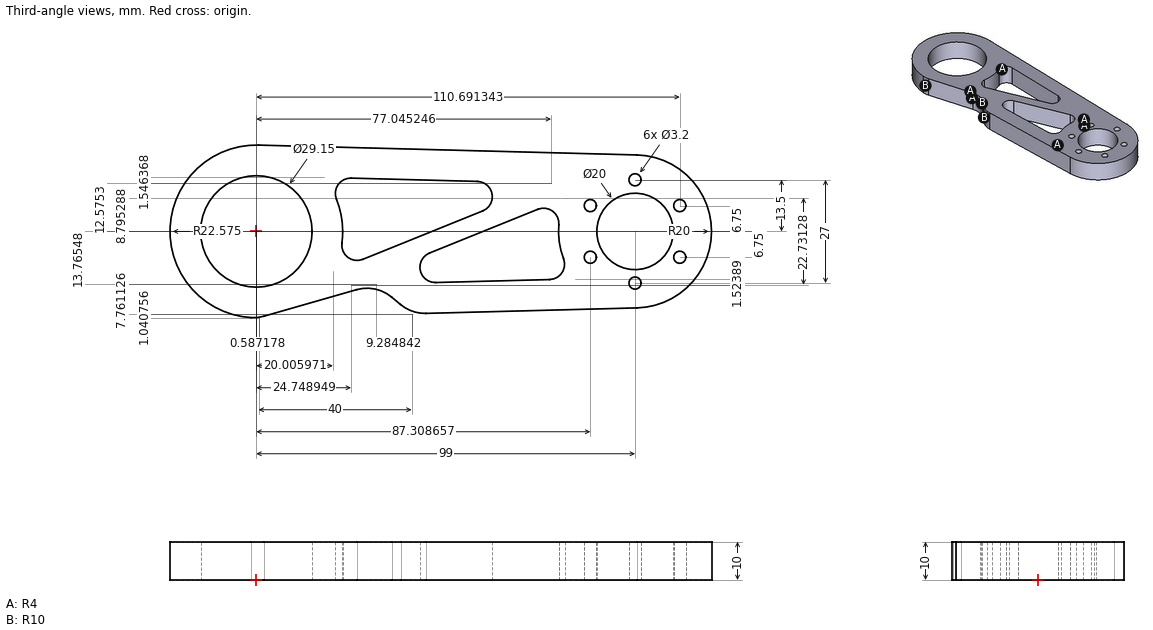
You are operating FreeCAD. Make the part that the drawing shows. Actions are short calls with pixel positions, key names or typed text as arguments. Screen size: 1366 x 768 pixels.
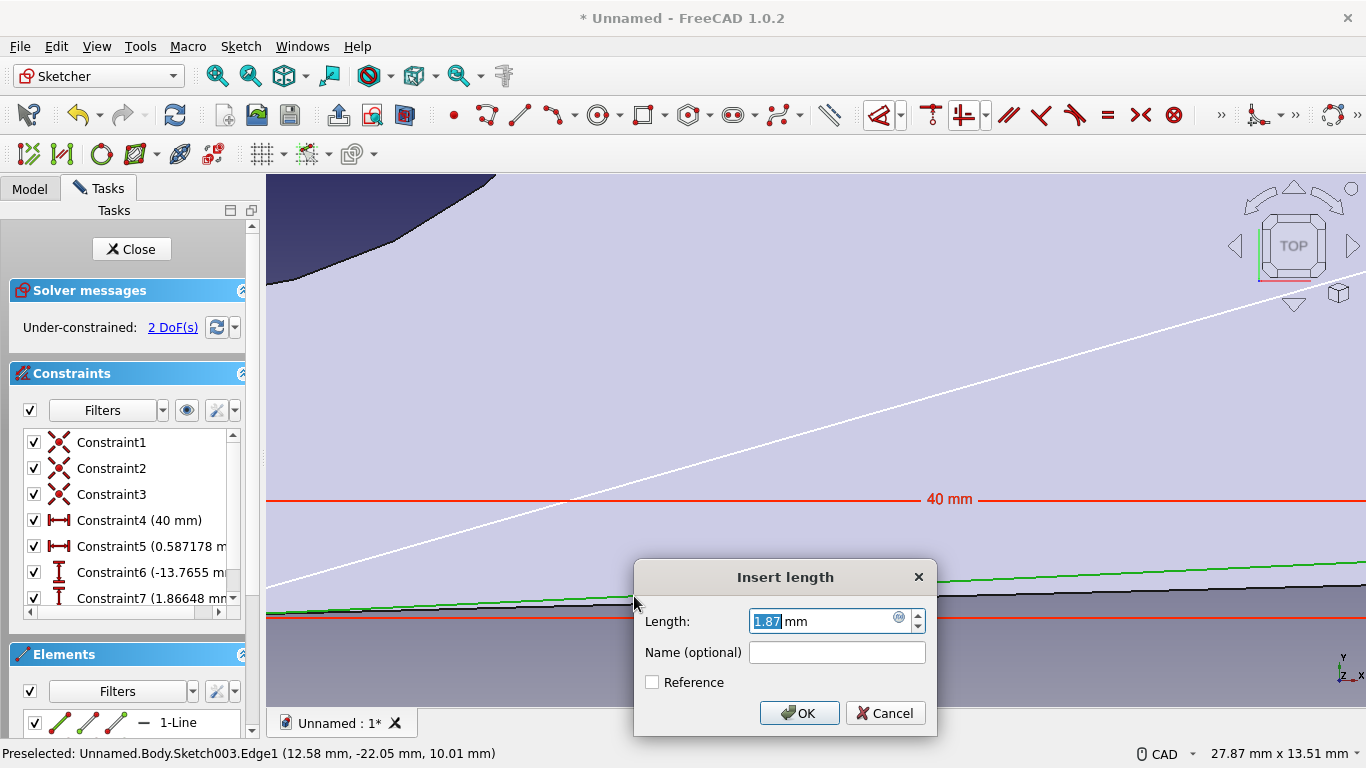
text(1.040756)
key(Return)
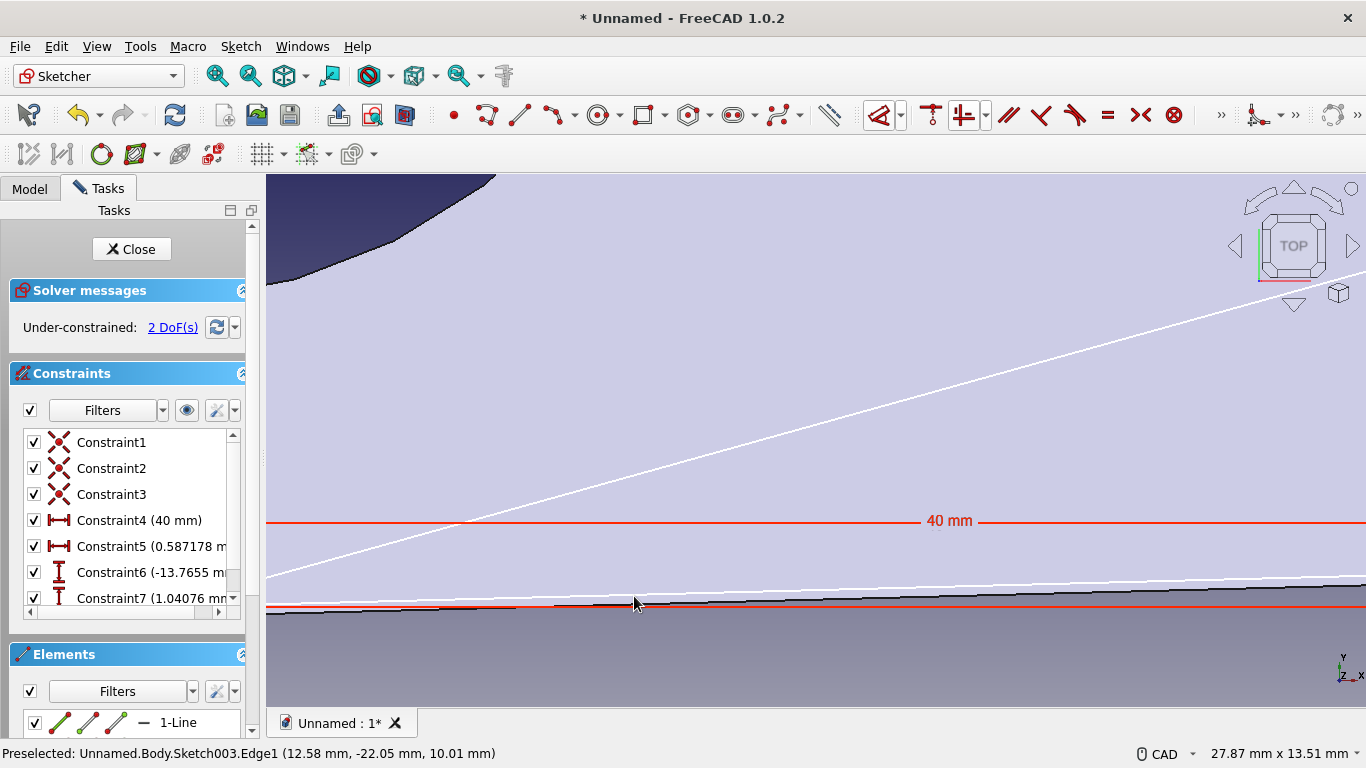
scroll(636, 597, down, 5)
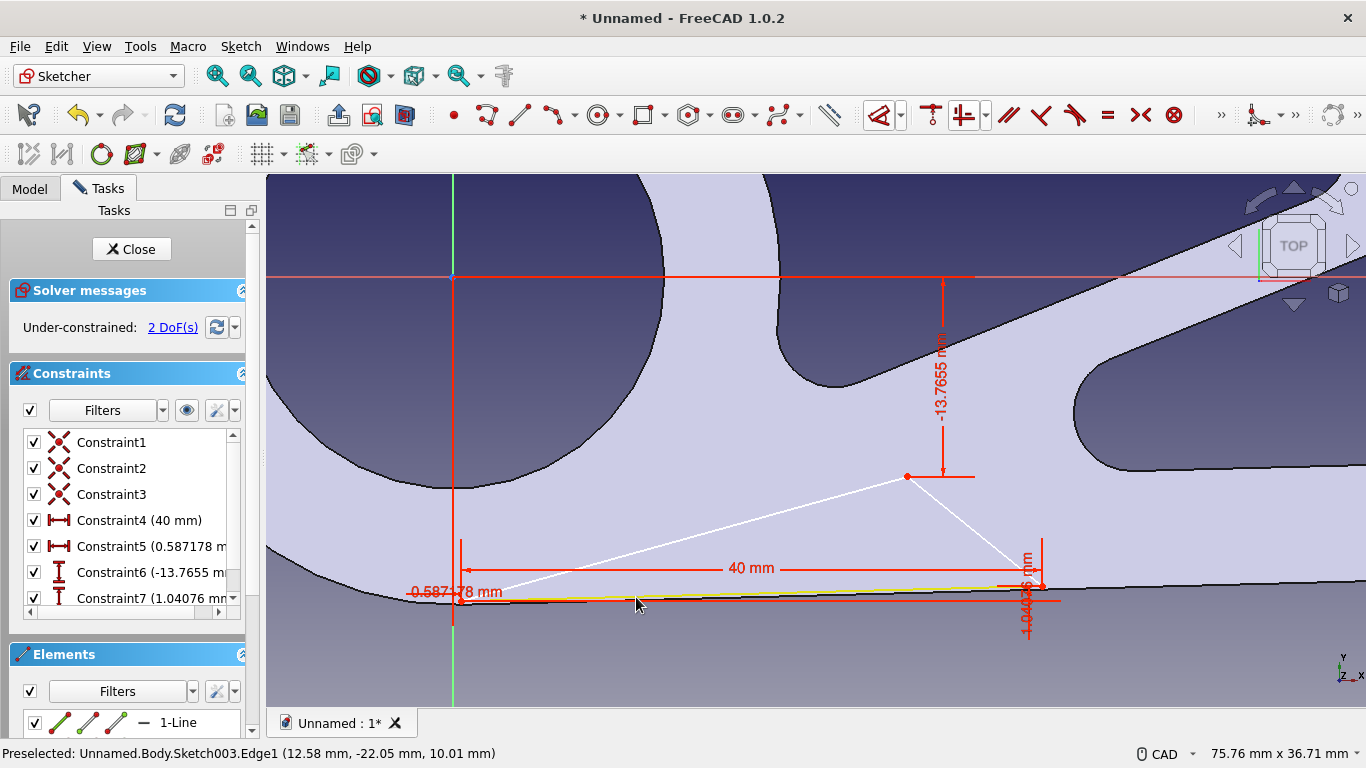
click(1002, 553)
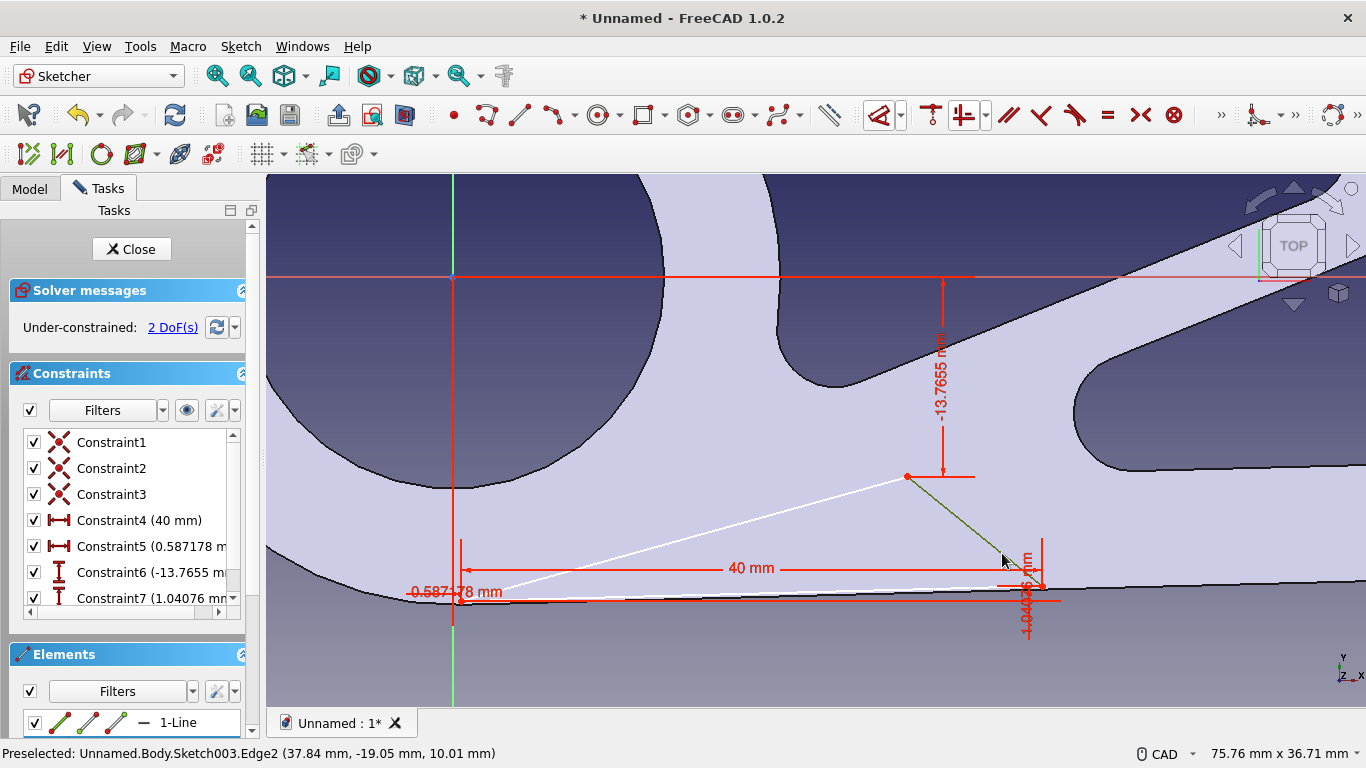
key(l)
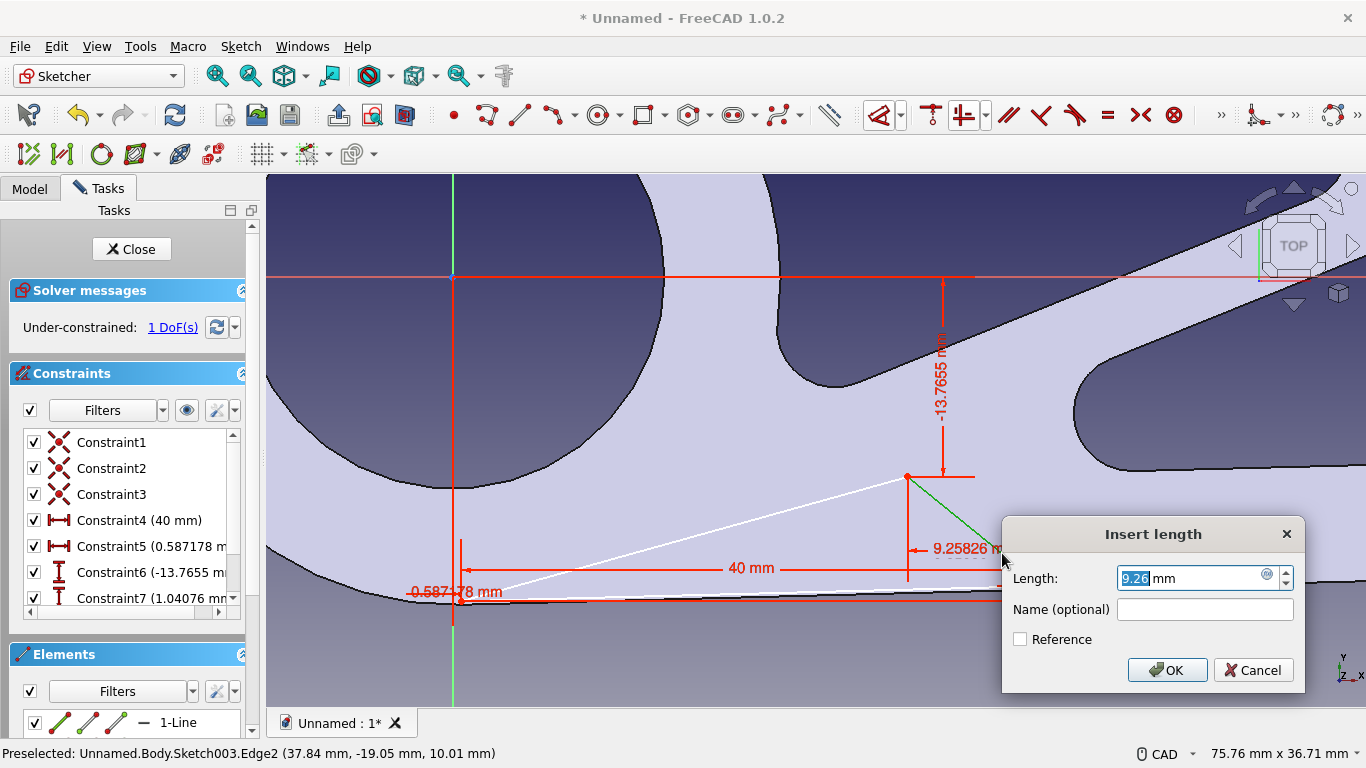
text(9.284842)
key(Return)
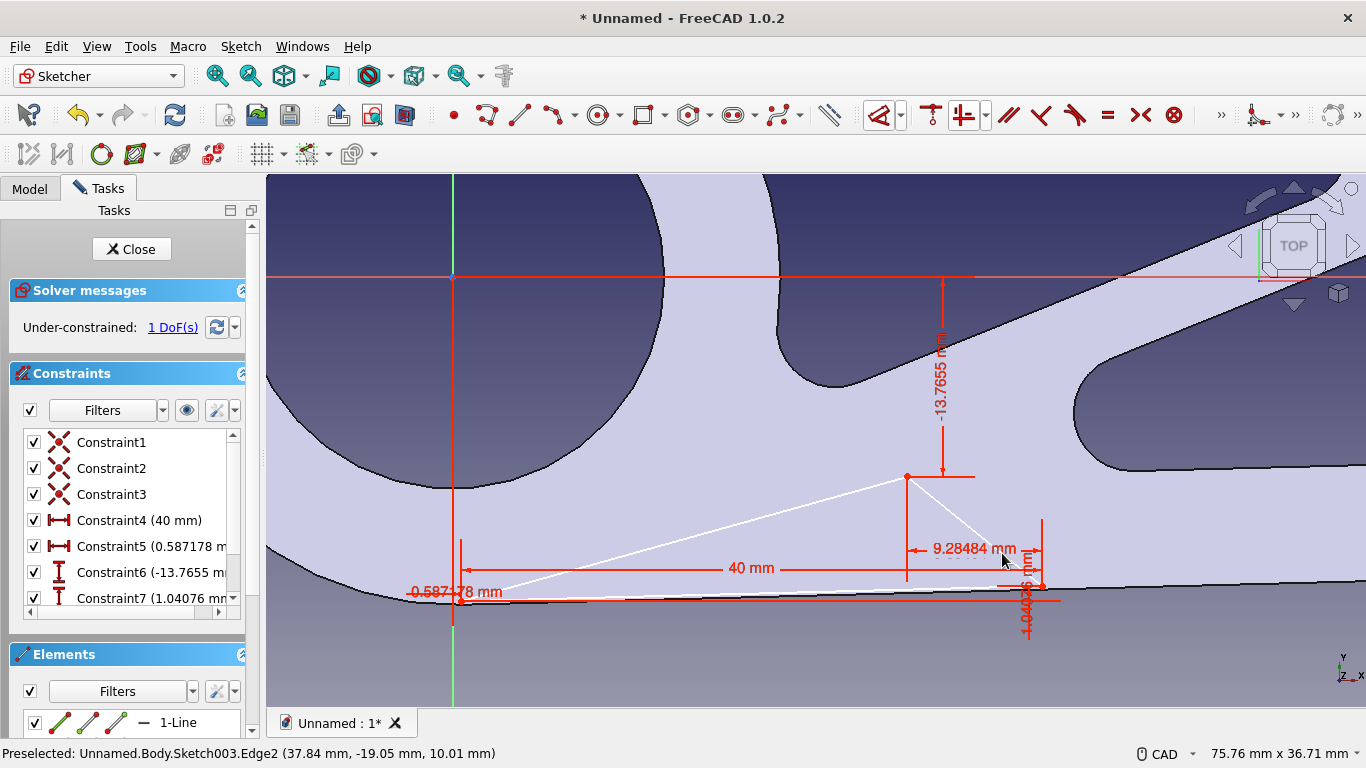
click(948, 510)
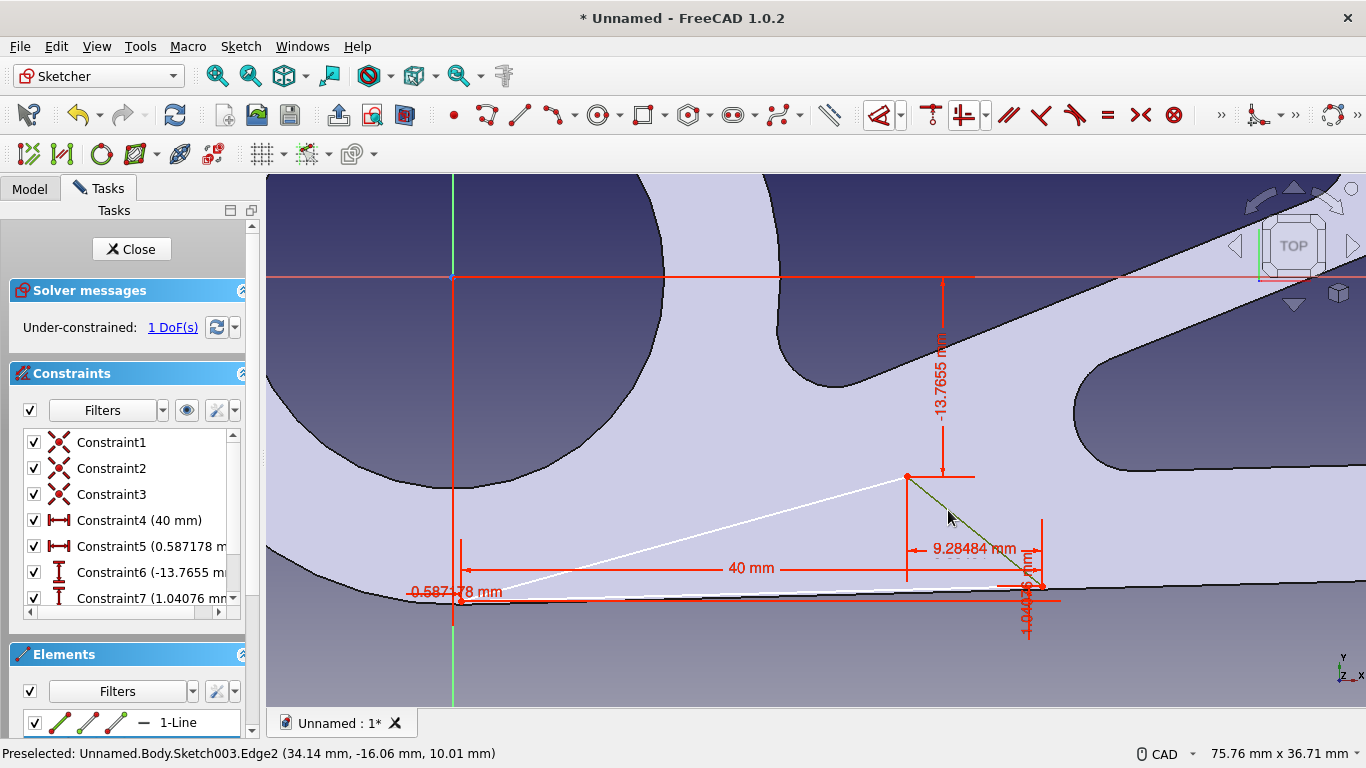
key(i)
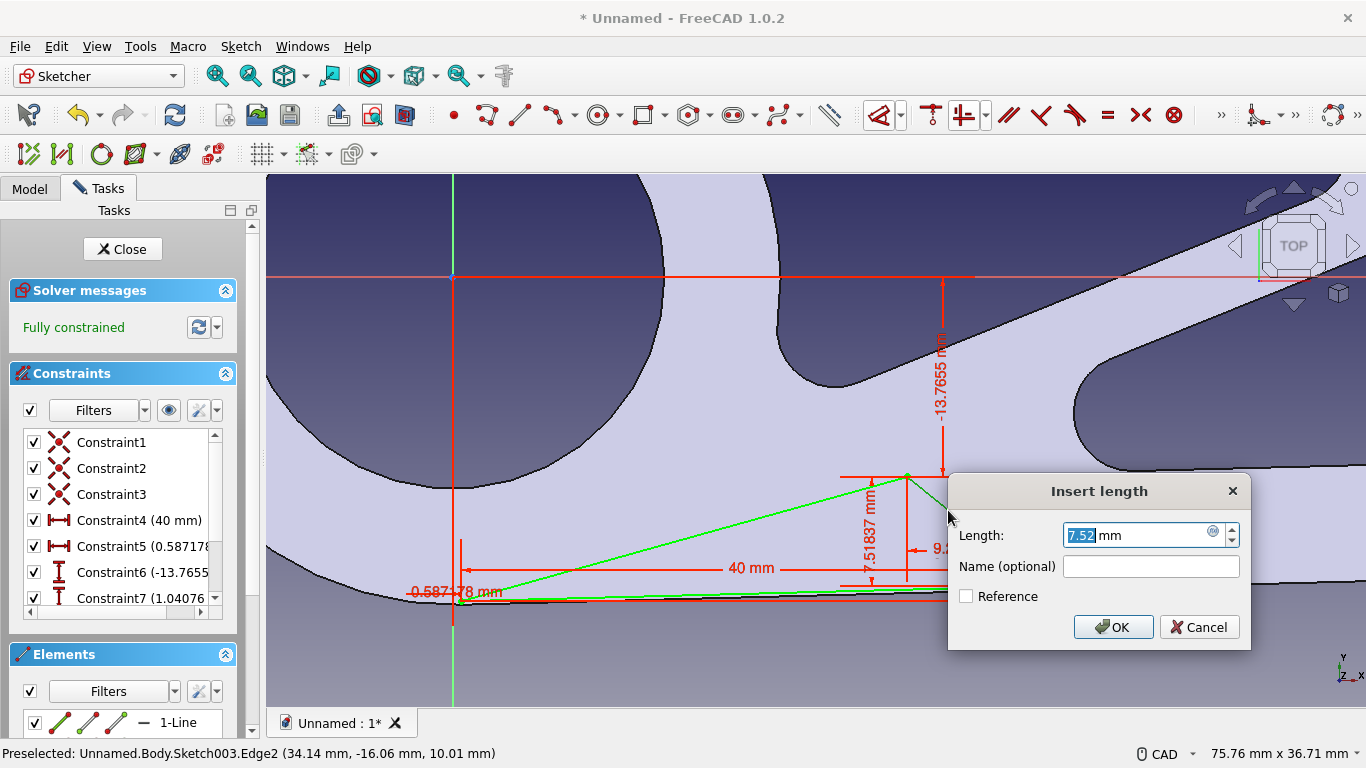
text(7.761126)
key(Return)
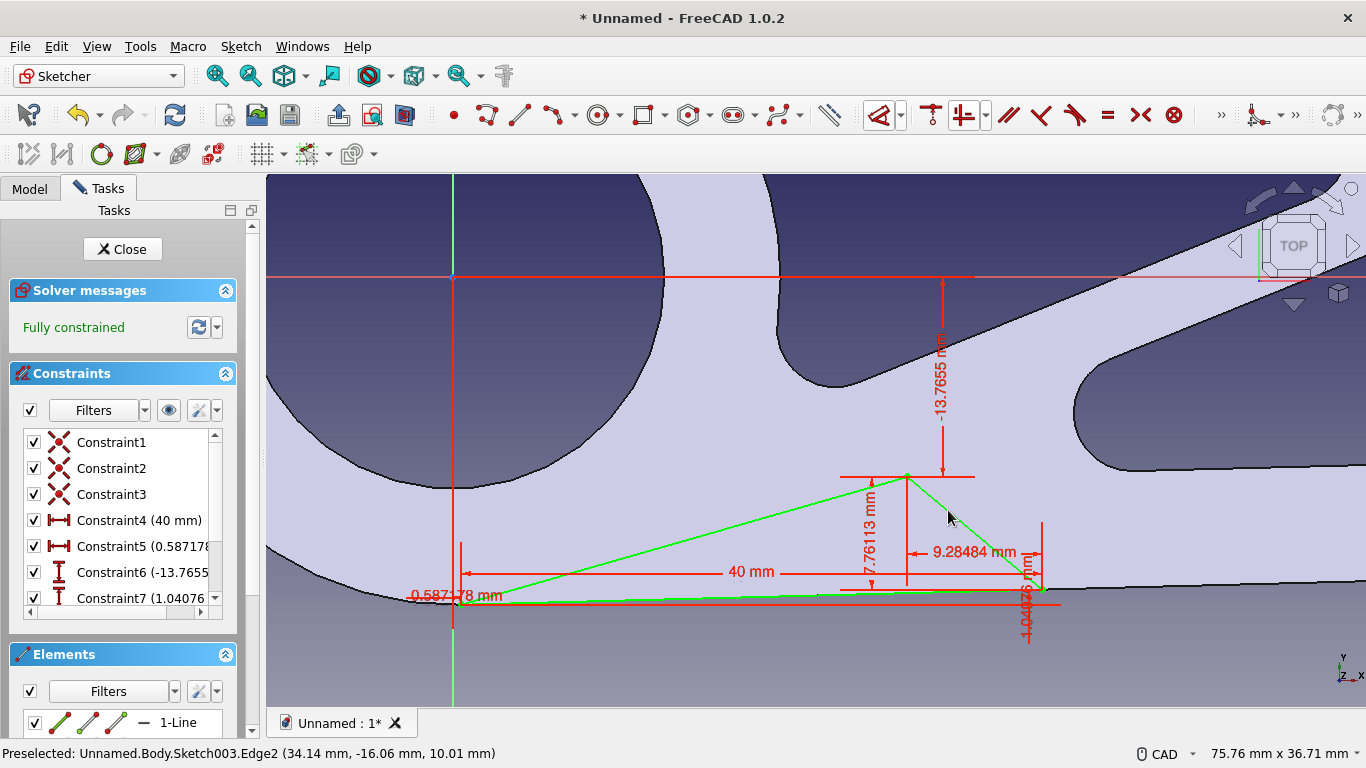
click(123, 249)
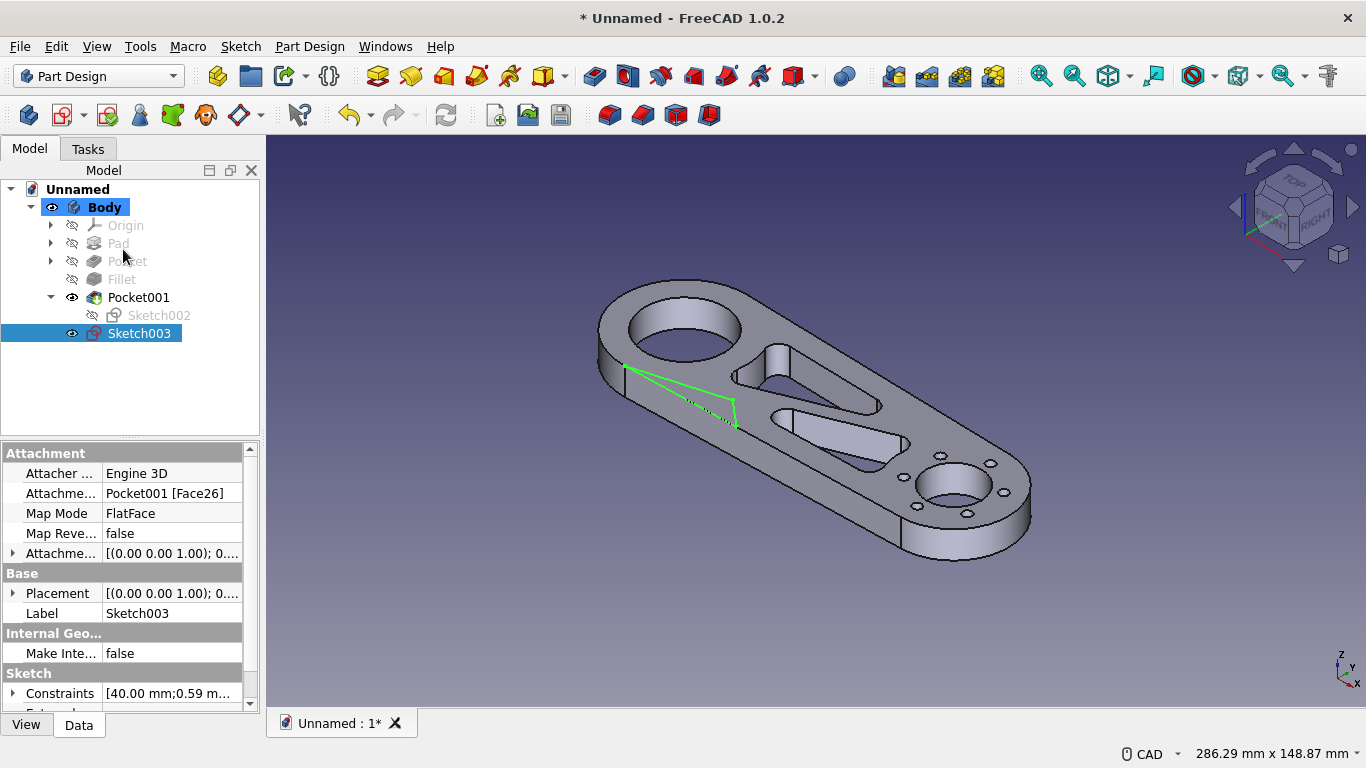
click(595, 76)